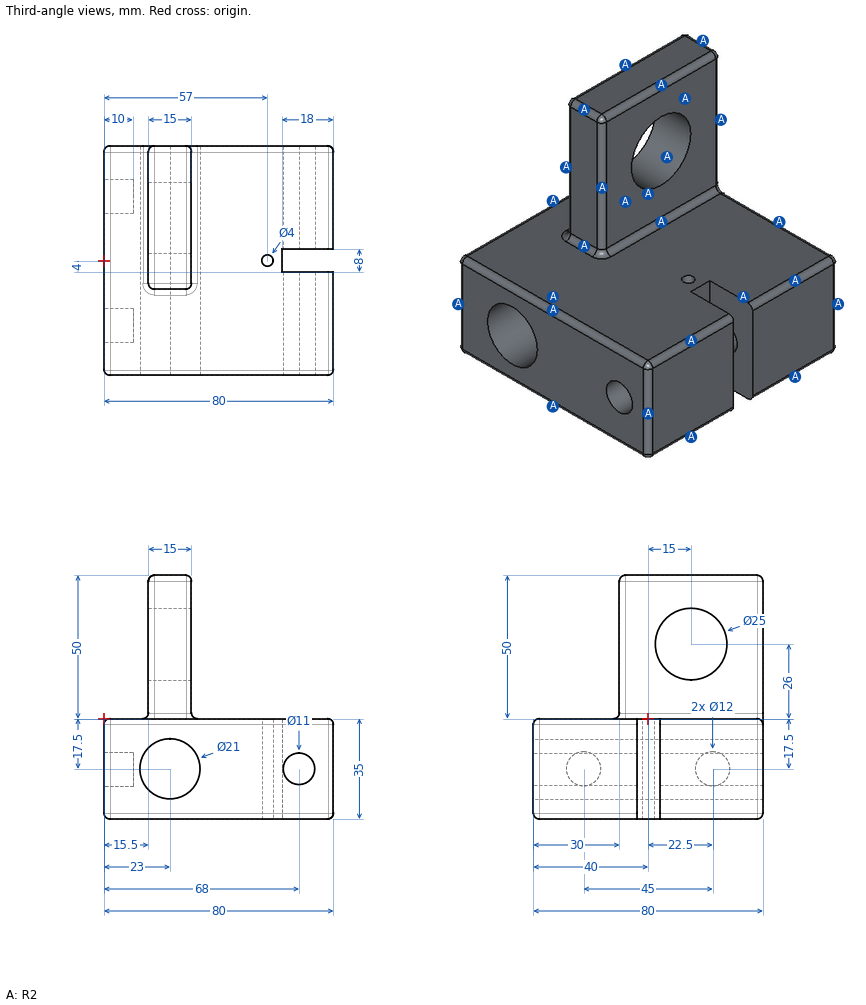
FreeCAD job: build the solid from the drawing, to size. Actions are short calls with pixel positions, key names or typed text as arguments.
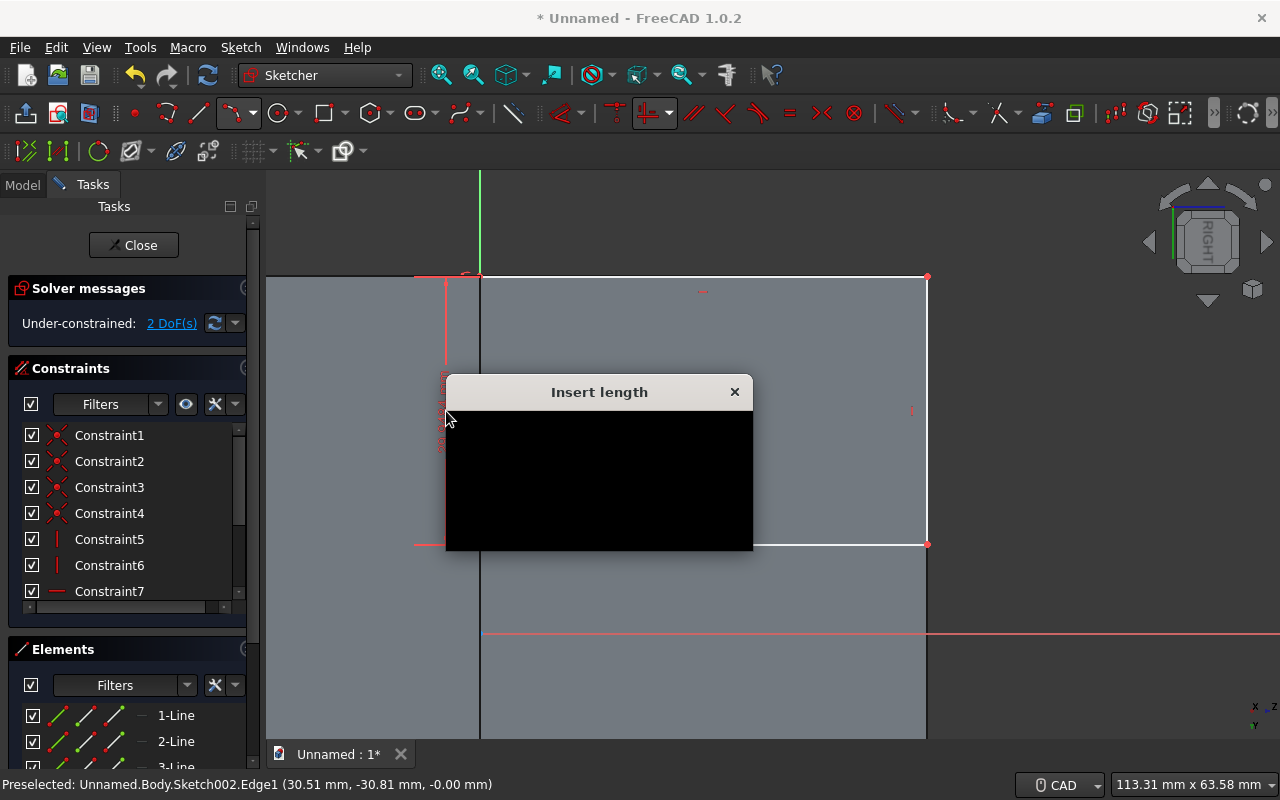
text(30)
key(Return)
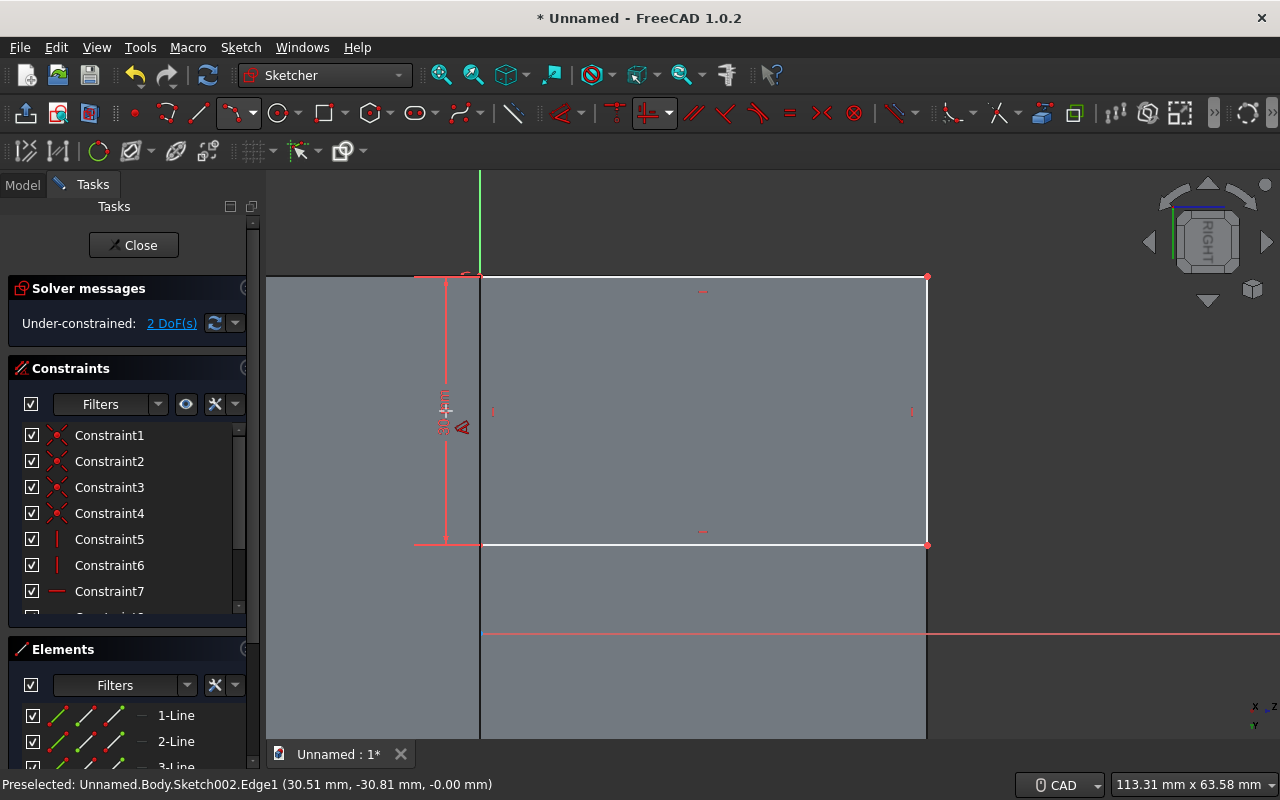
click(614, 545)
click(703, 579)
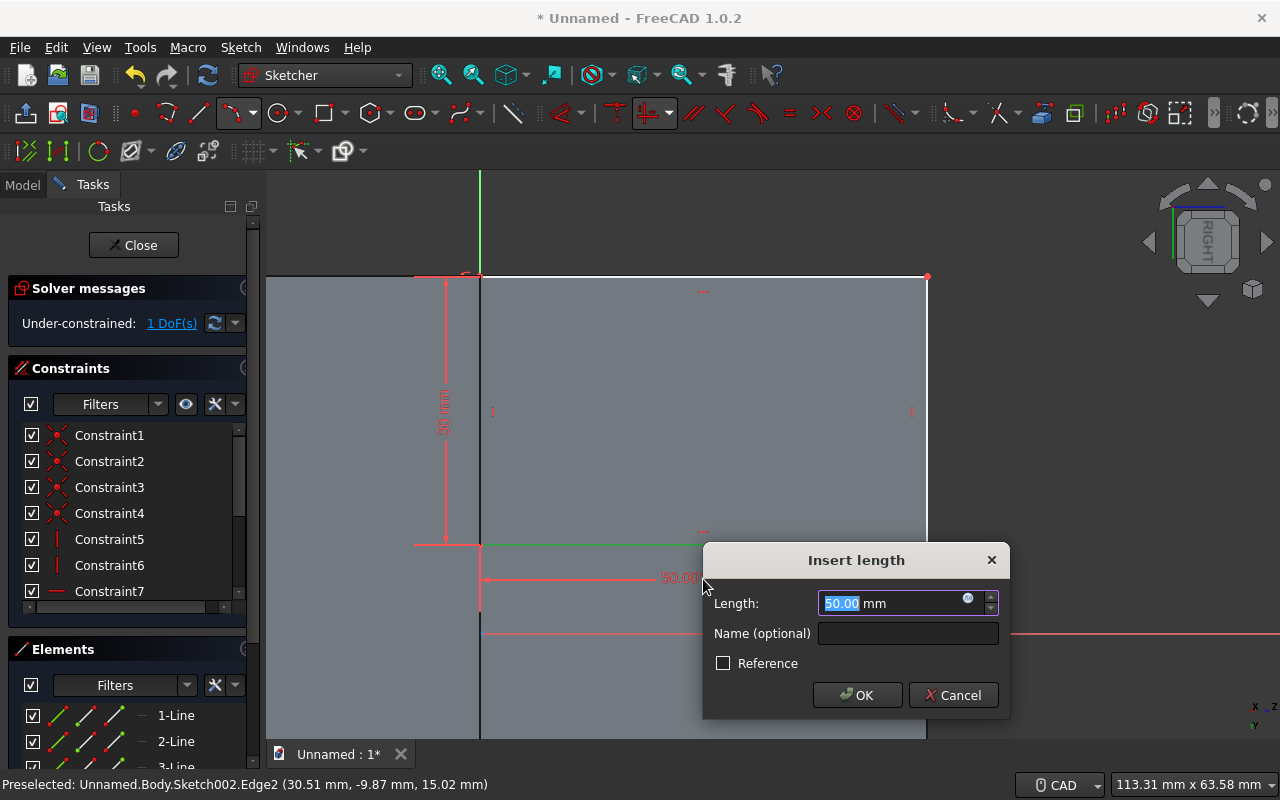
text(50)
key(Return)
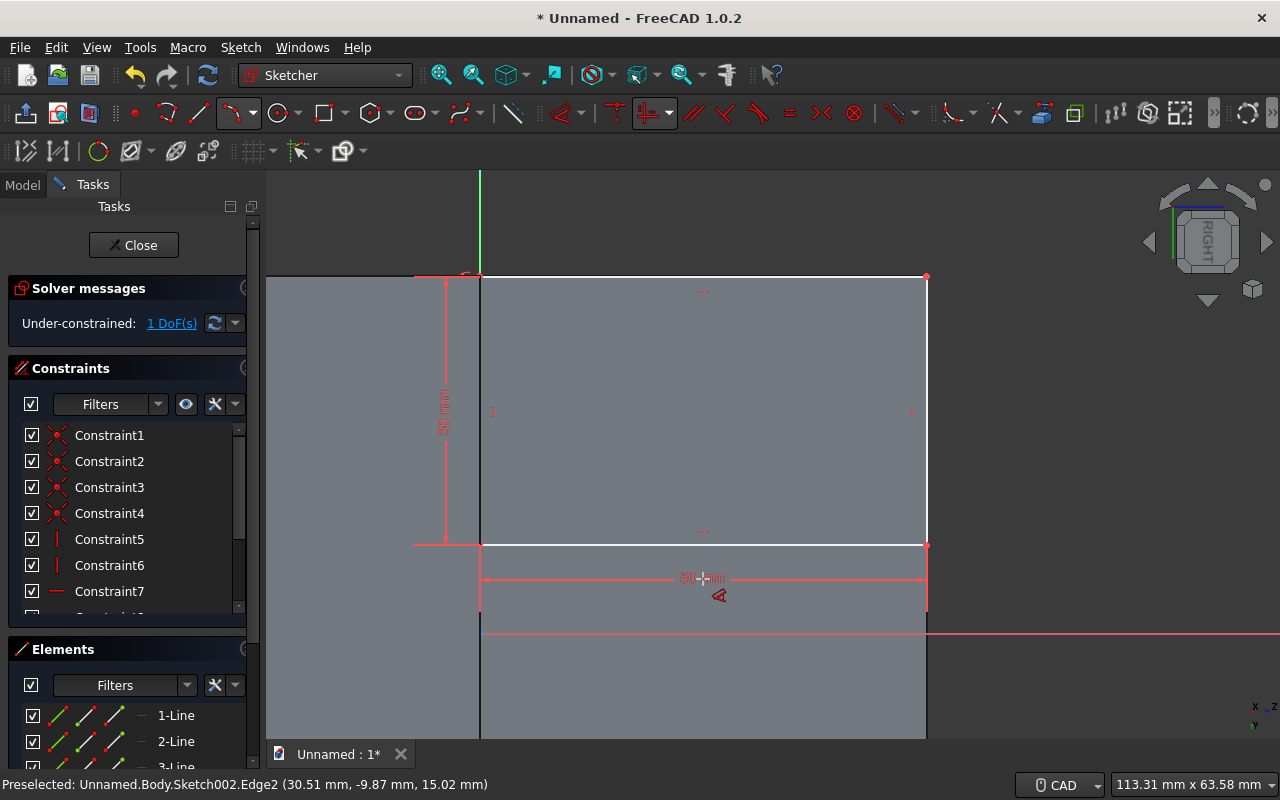
click(480, 277)
click(446, 455)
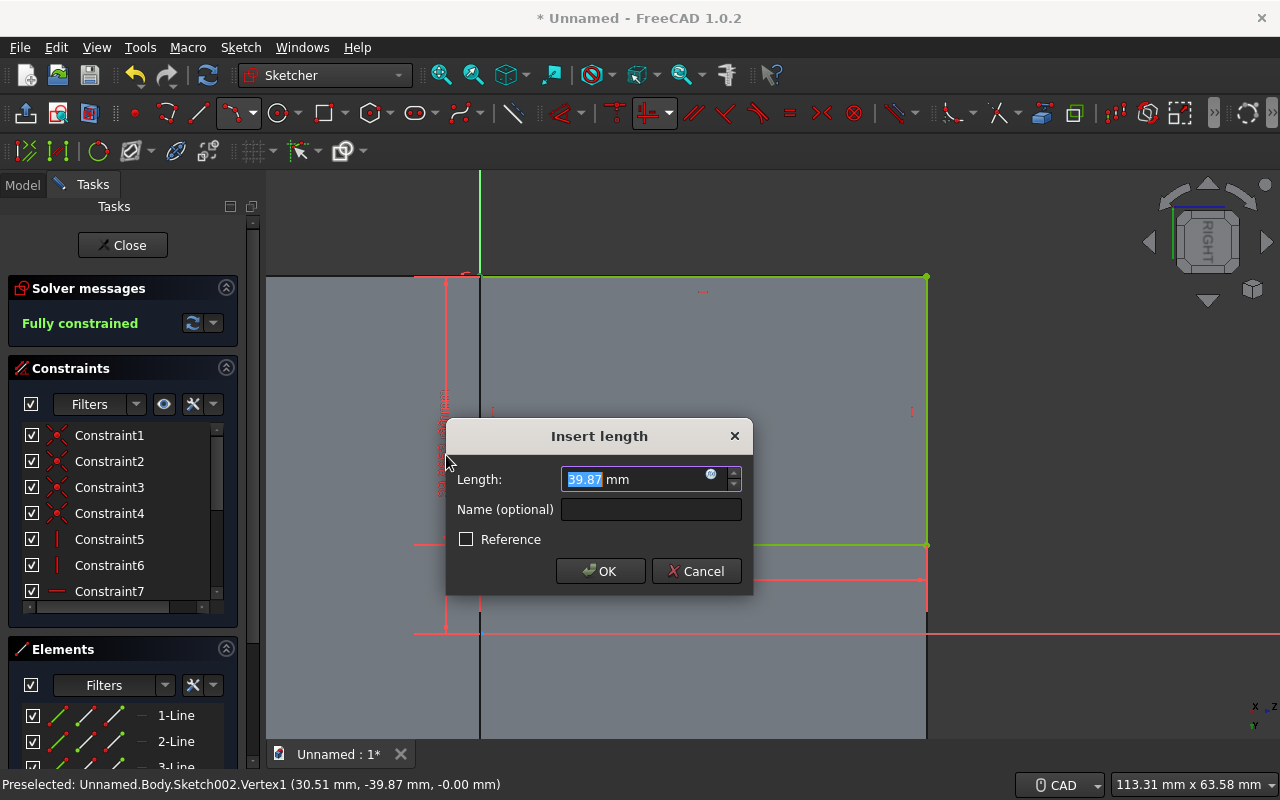
text(40)
key(Return)
key(Escape)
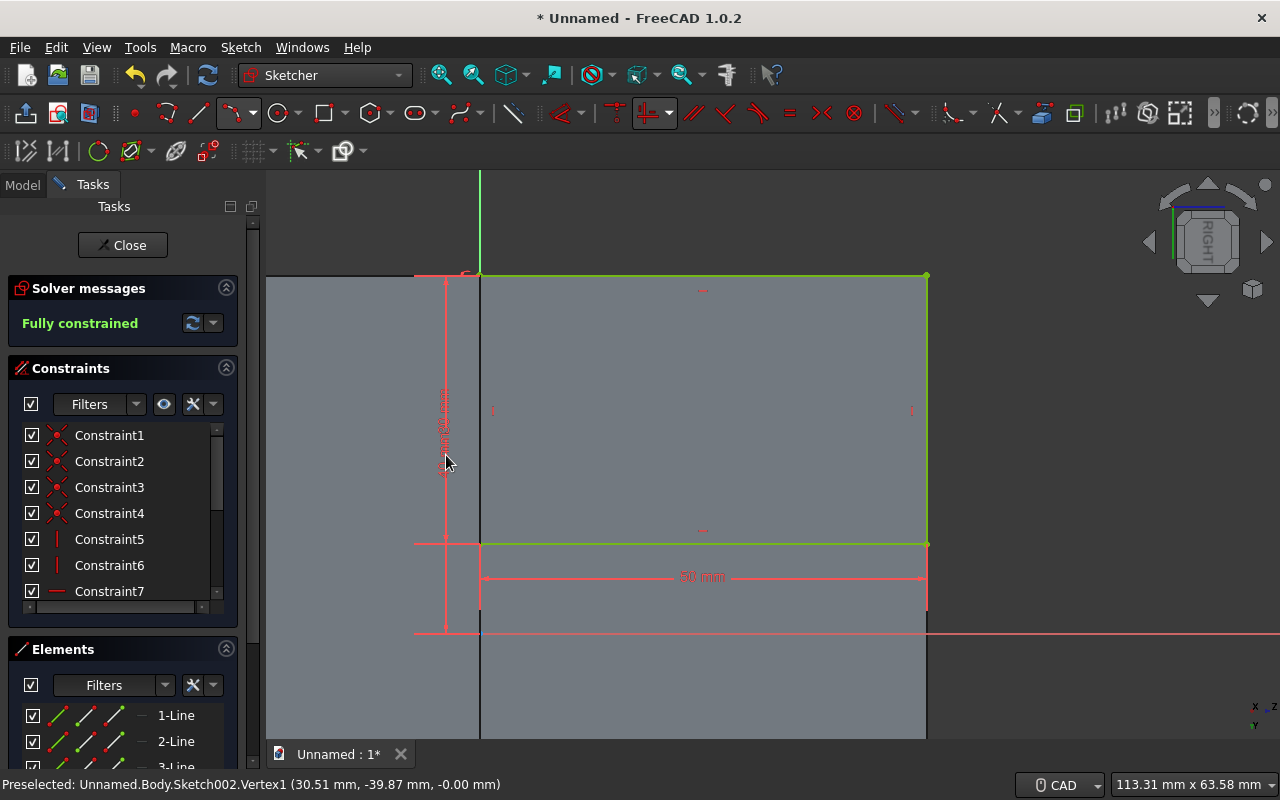
click(123, 245)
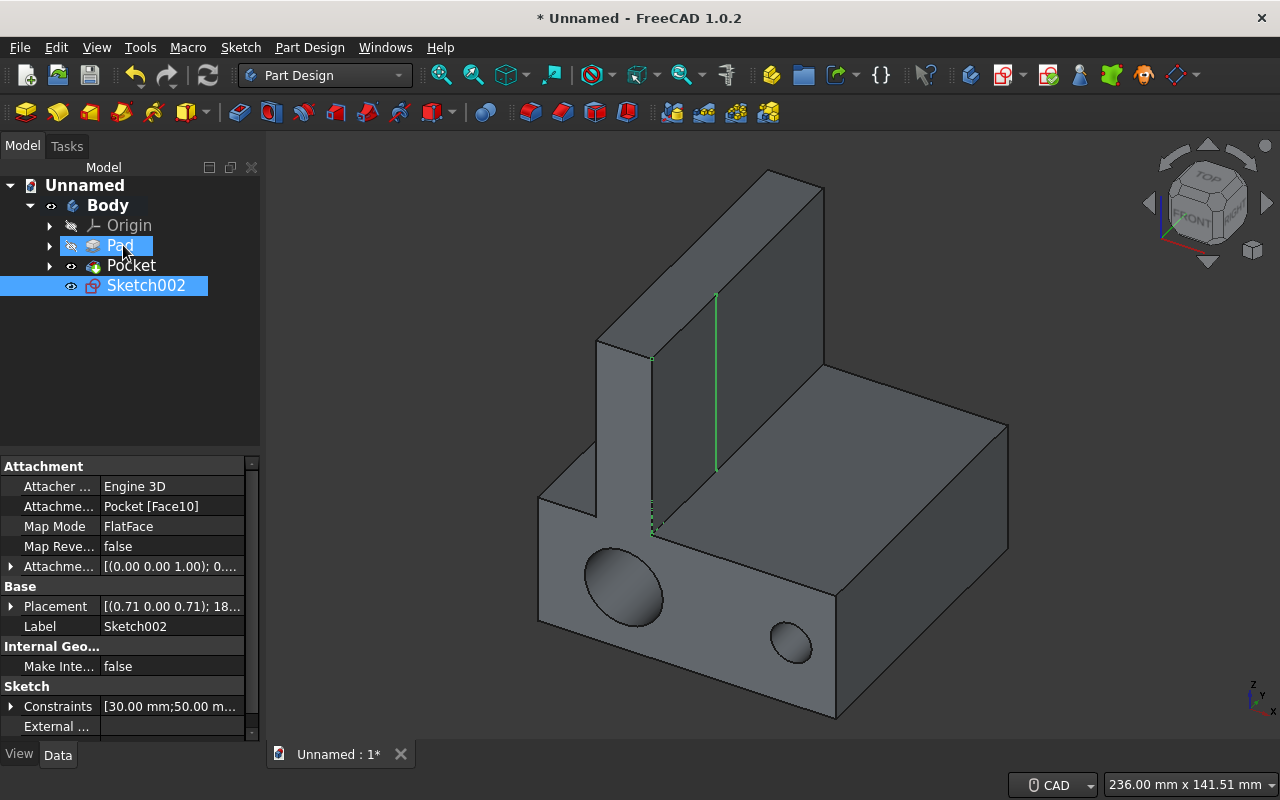
click(240, 112)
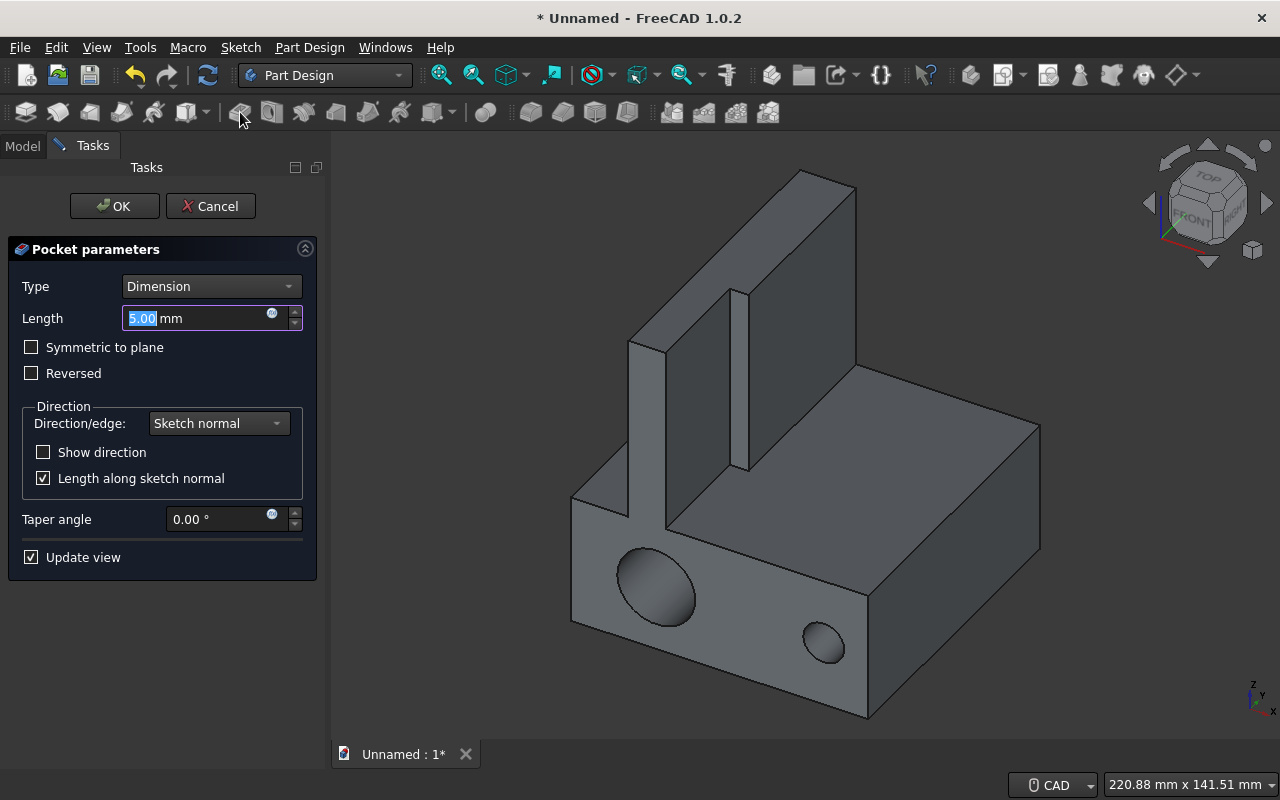
click(212, 286)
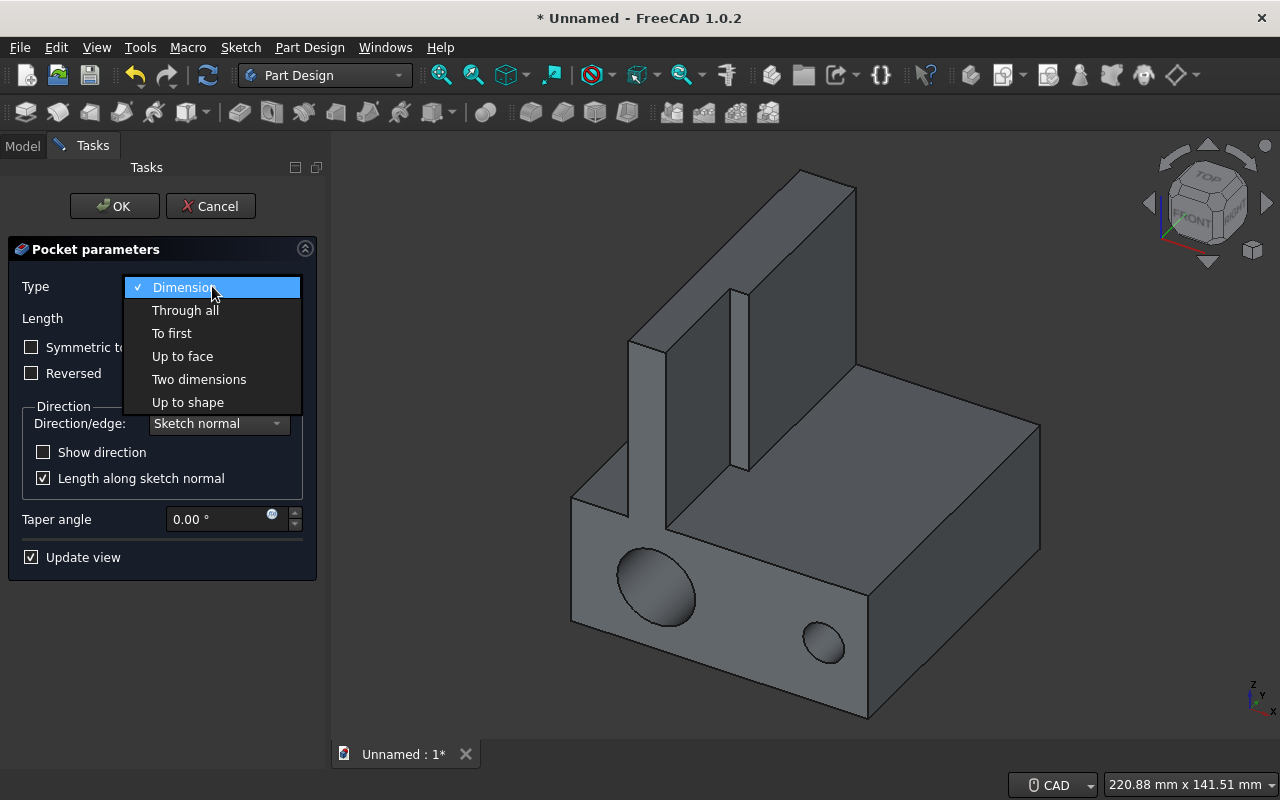
click(212, 310)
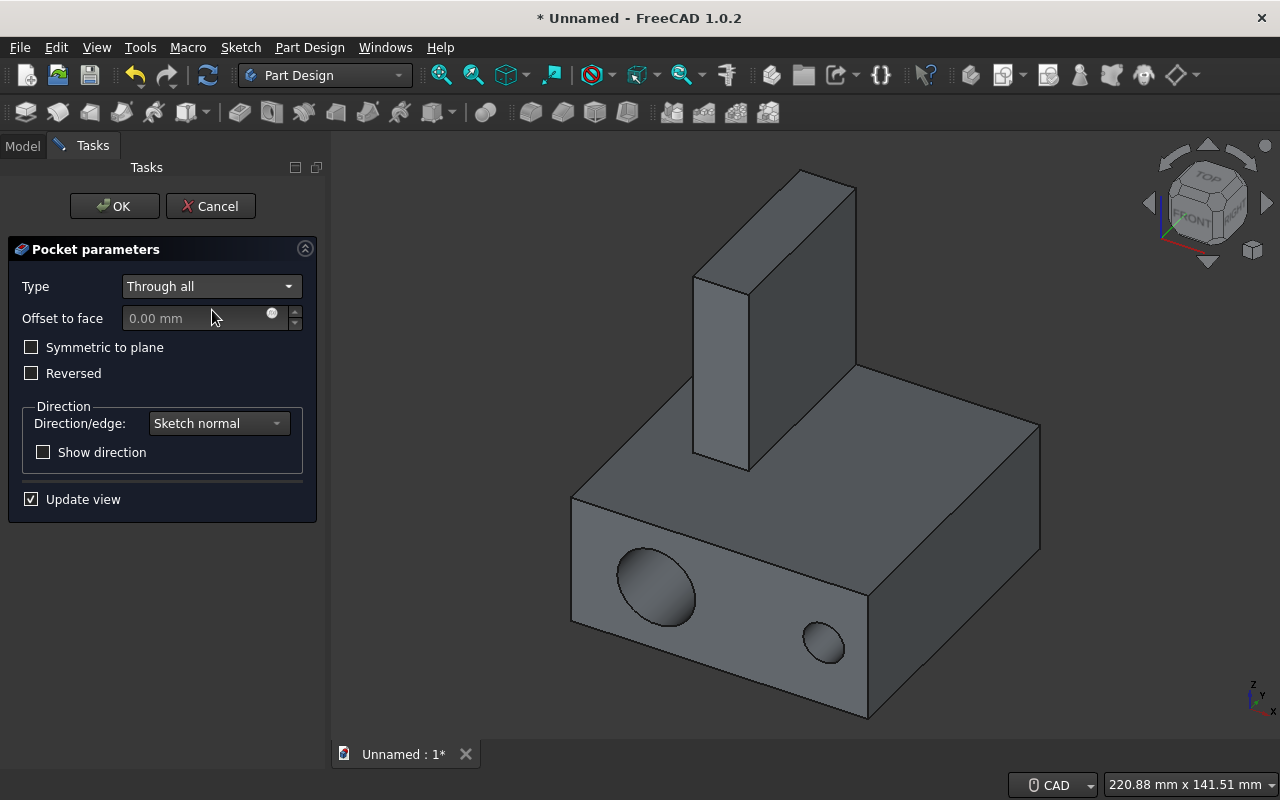
click(115, 206)